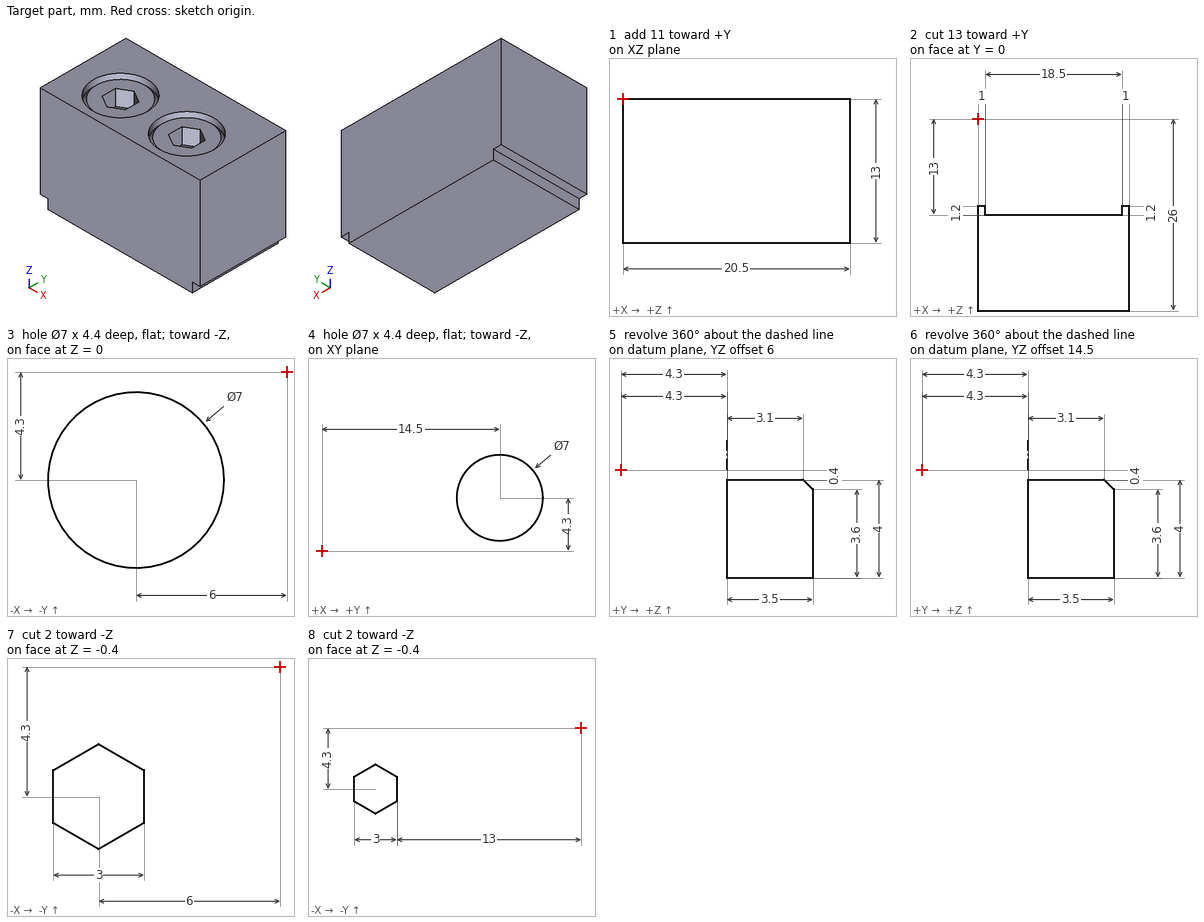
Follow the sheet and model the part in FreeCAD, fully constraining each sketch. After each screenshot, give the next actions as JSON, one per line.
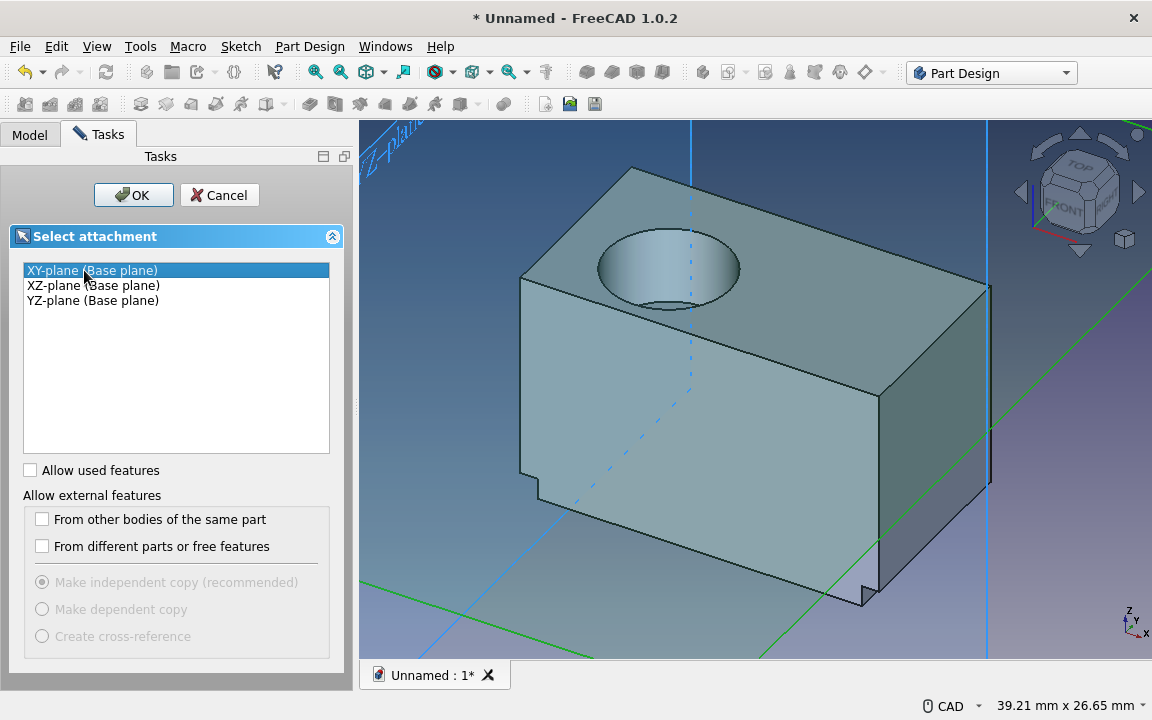
{"action": "left_click", "coordinate": [134, 195]}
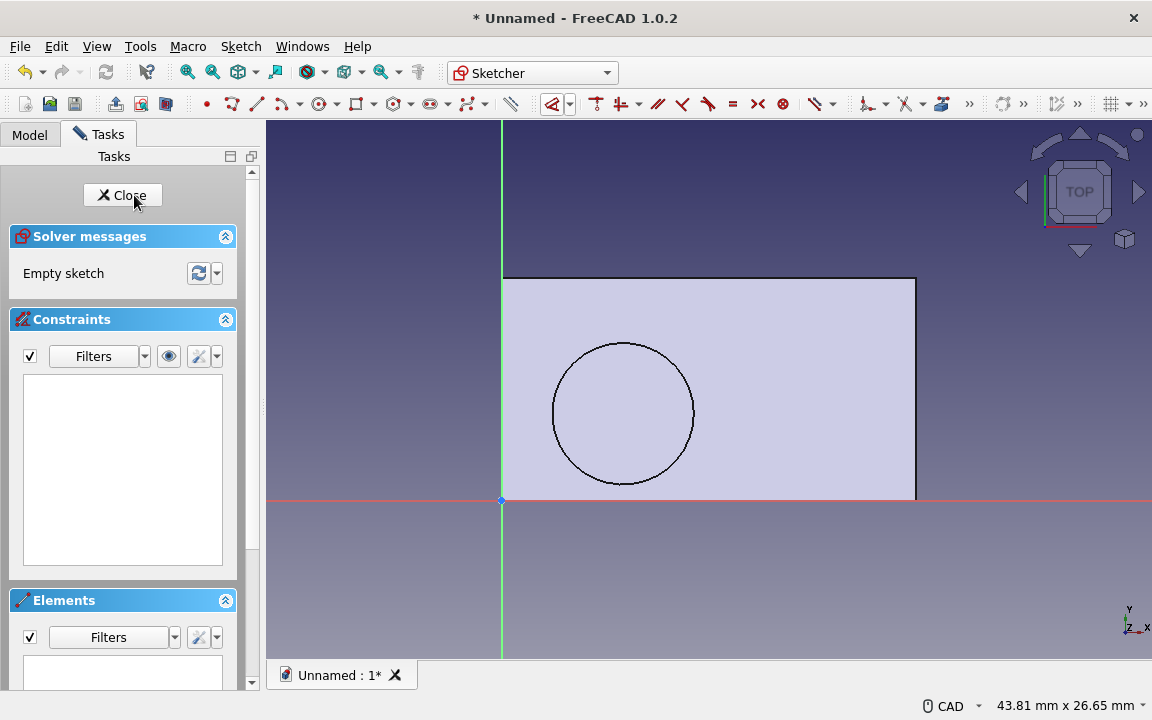
{"action": "scroll", "coordinate": [921, 434], "scroll_direction": "up", "scroll_amount": 4}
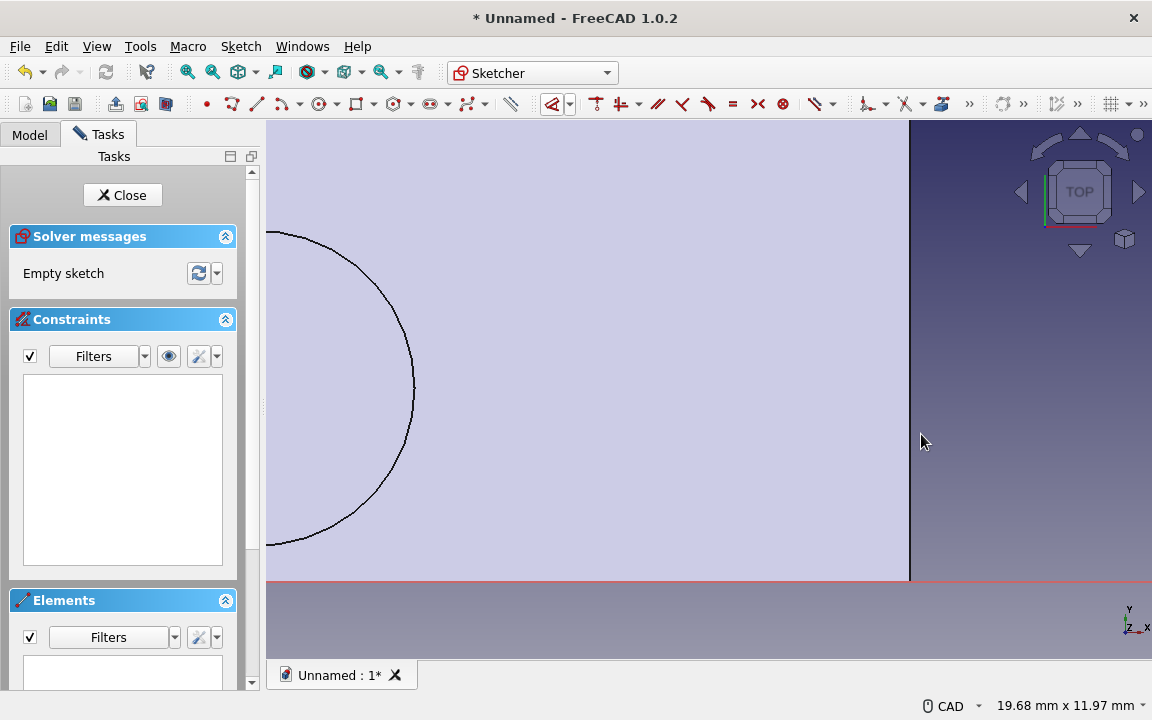
{"action": "key", "text": "g c"}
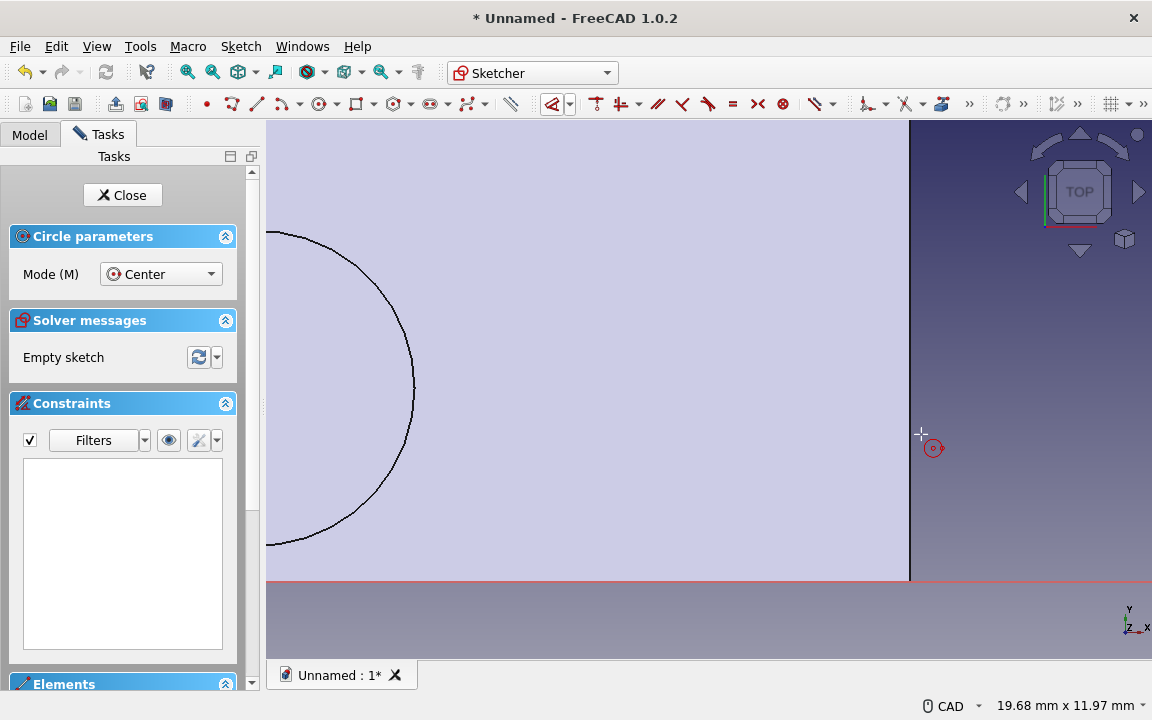
{"action": "left_click", "coordinate": [640, 388]}
{"action": "mouse_move", "coordinate": [751, 277]}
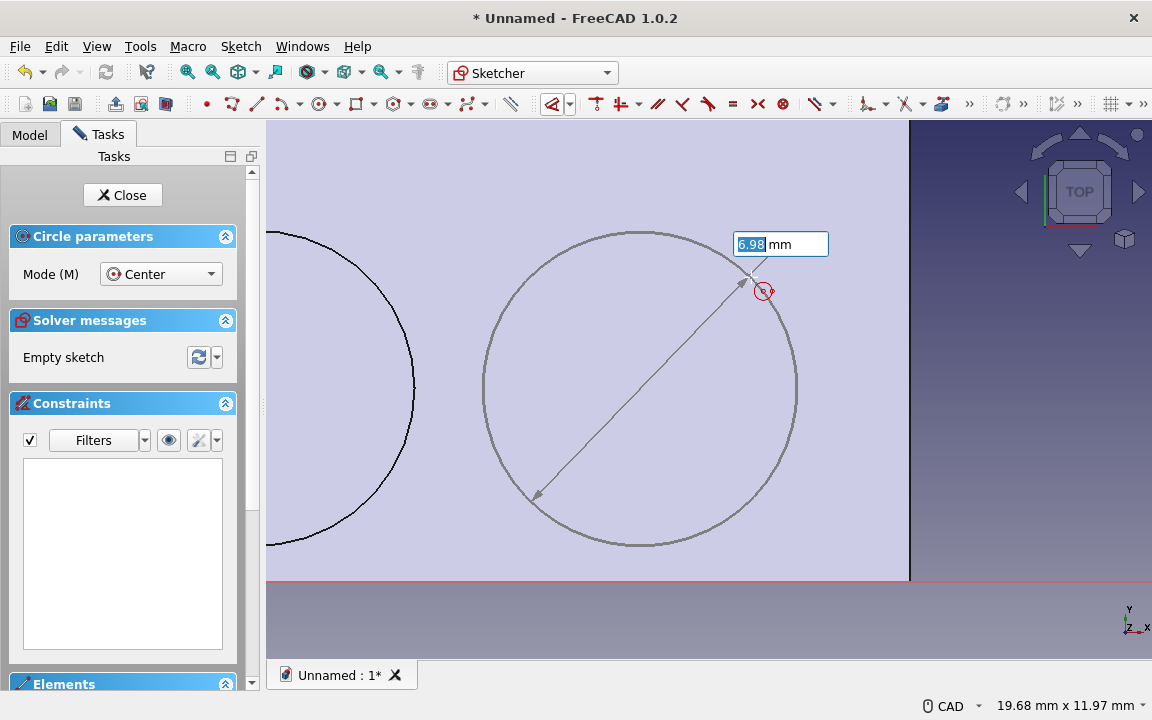
{"action": "type", "text": "7"}
{"action": "key", "text": "Return"}
{"action": "key", "text": "Escape"}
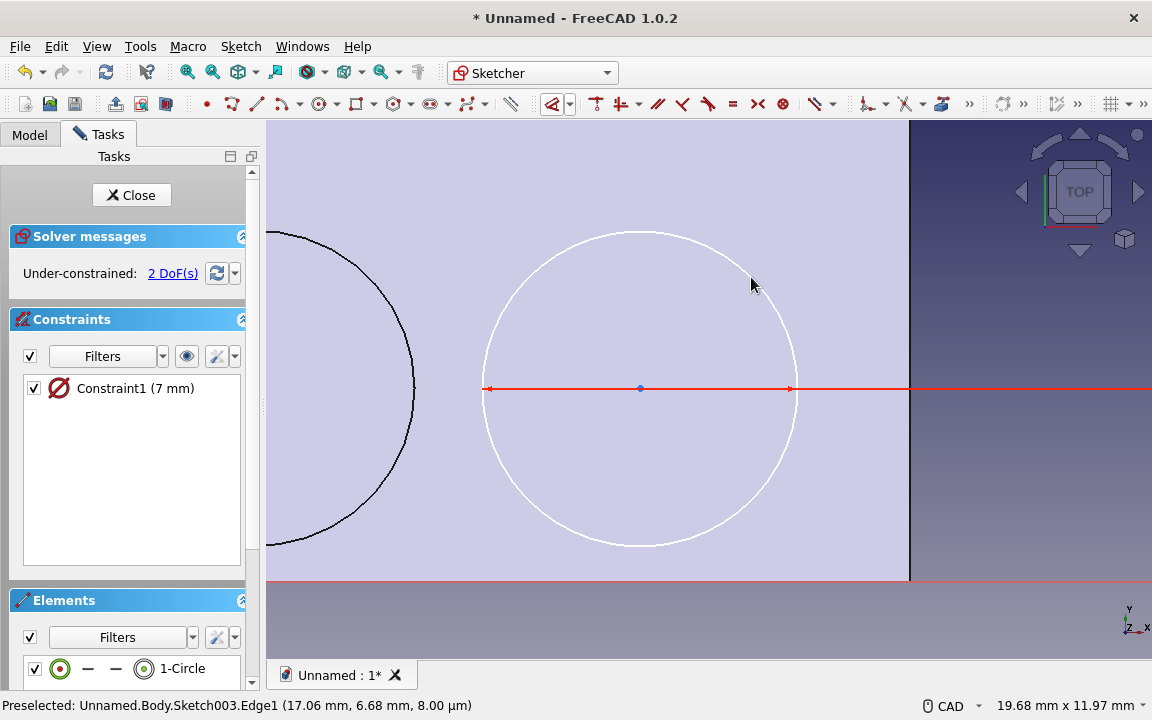
{"action": "left_click", "coordinate": [640, 389]}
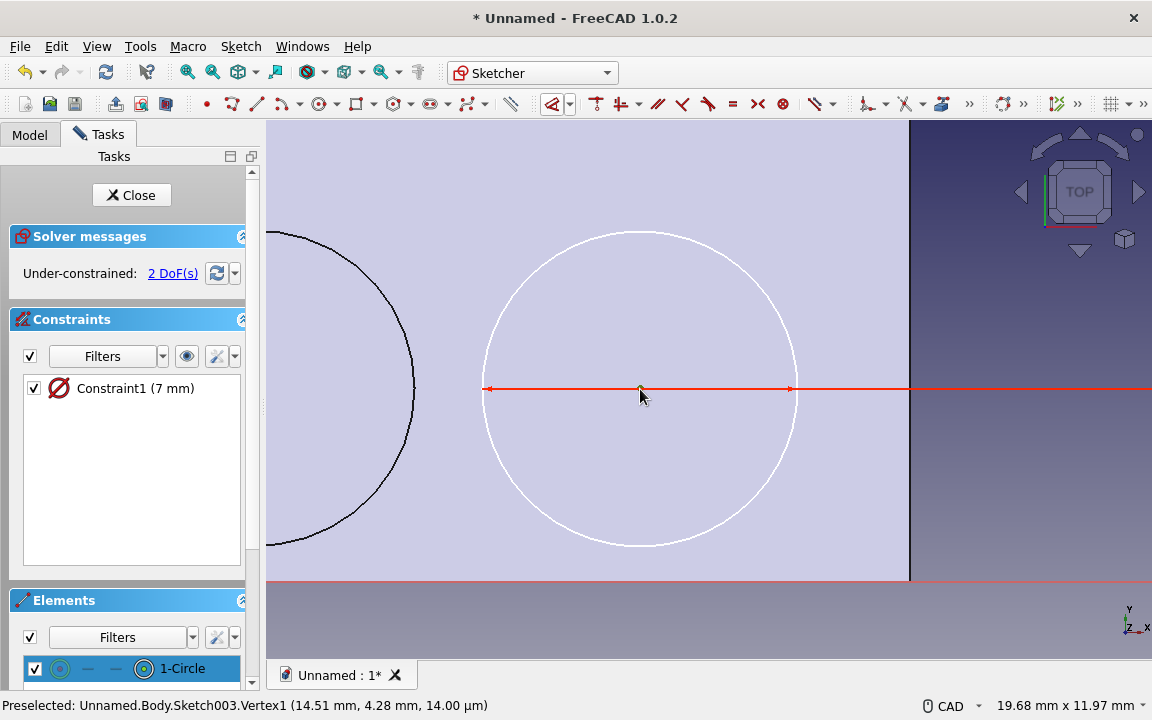
{"action": "left_click", "coordinate": [570, 104]}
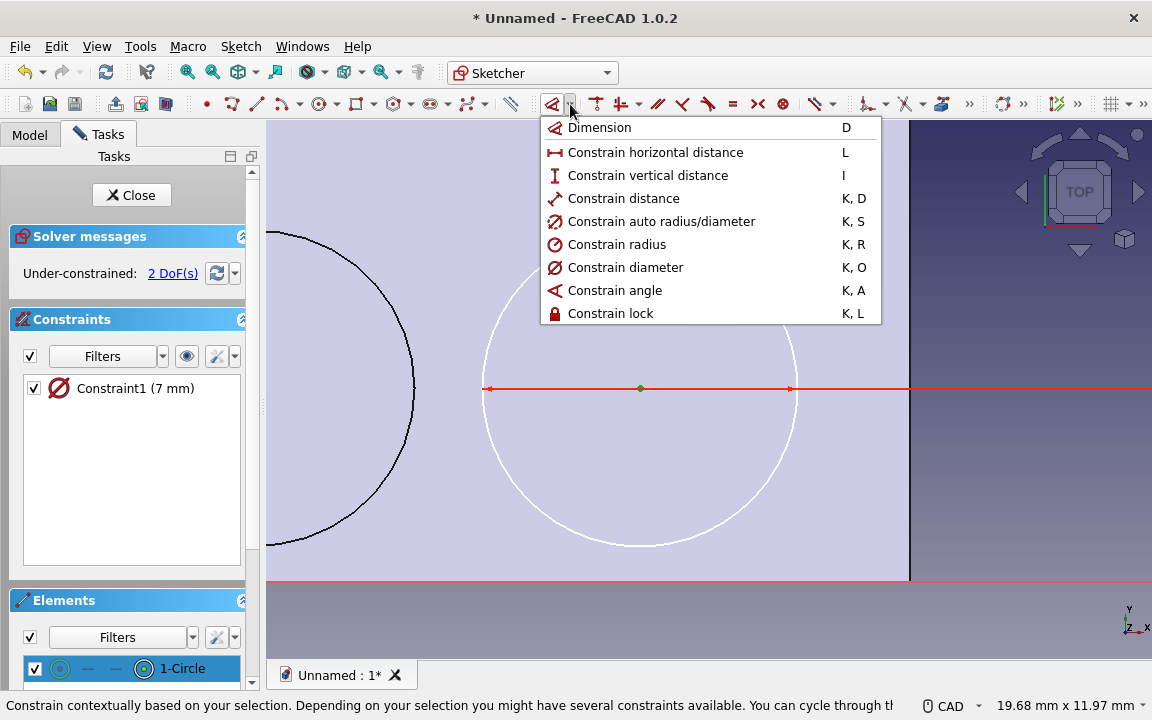
{"action": "left_click", "coordinate": [711, 176]}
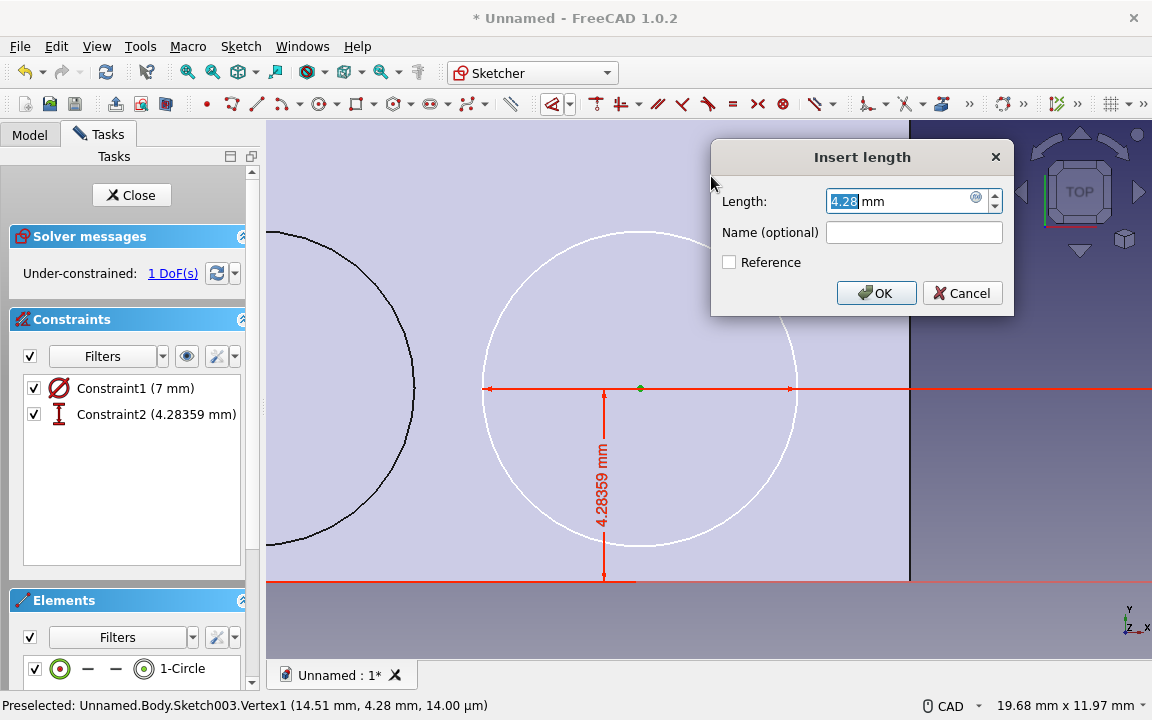
{"action": "type", "text": "4.3"}
{"action": "key", "text": "Return"}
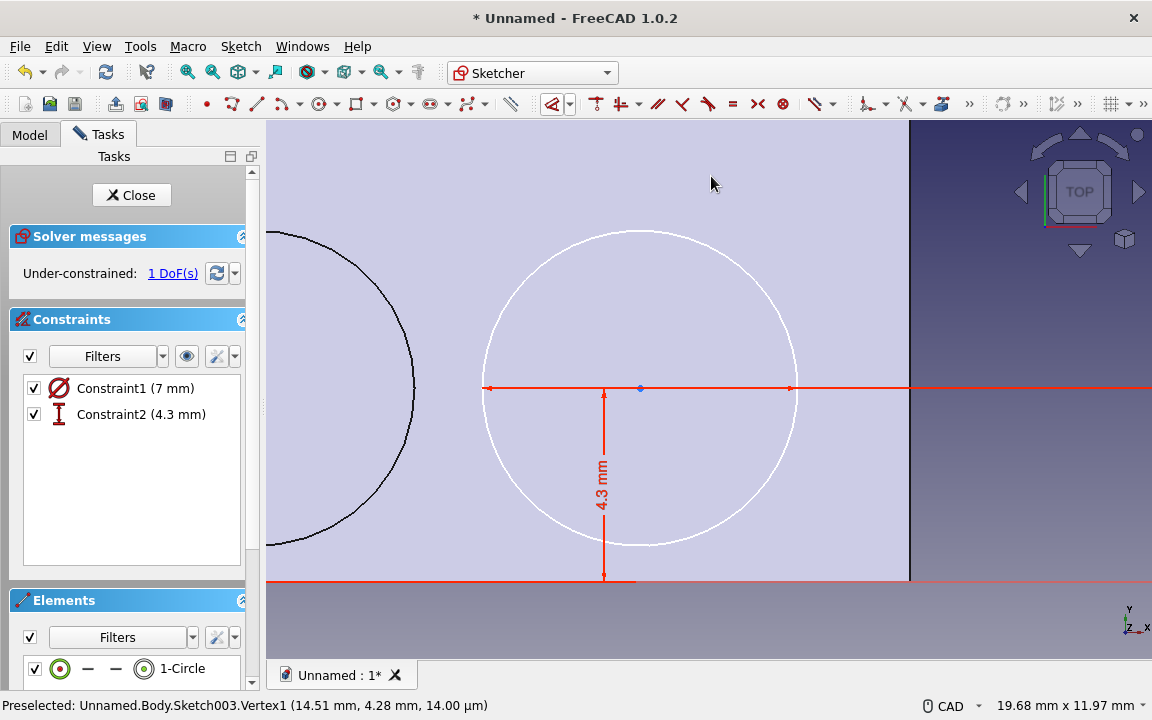
{"action": "left_click", "coordinate": [640, 388]}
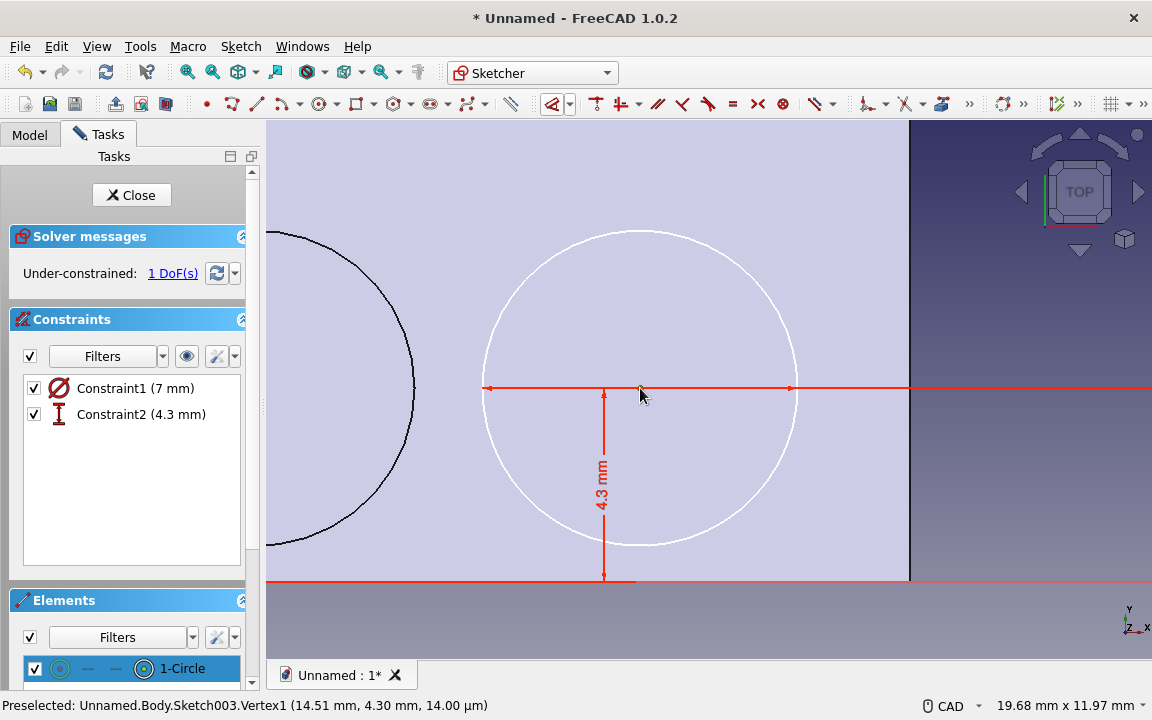
{"action": "left_click", "coordinate": [570, 104]}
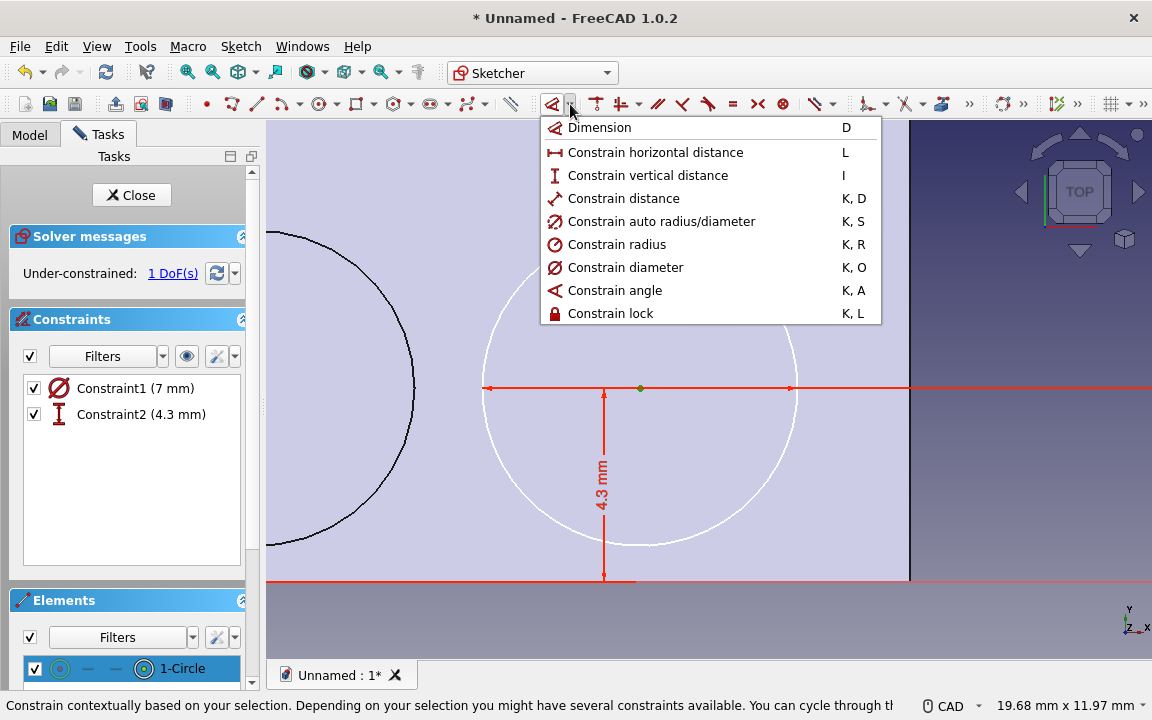
{"action": "left_click", "coordinate": [711, 152]}